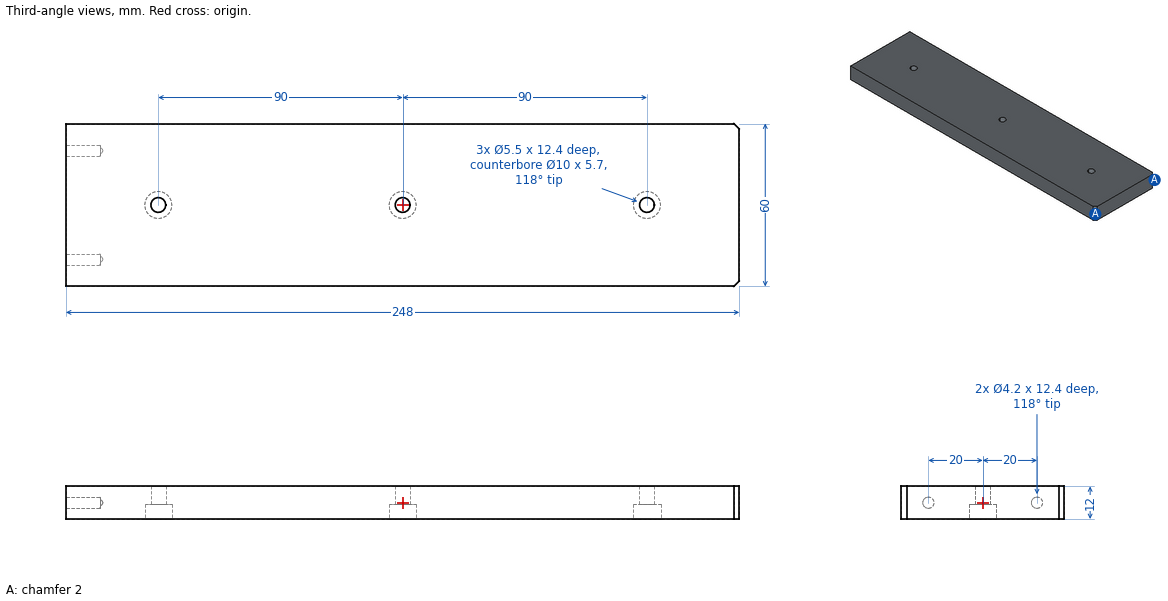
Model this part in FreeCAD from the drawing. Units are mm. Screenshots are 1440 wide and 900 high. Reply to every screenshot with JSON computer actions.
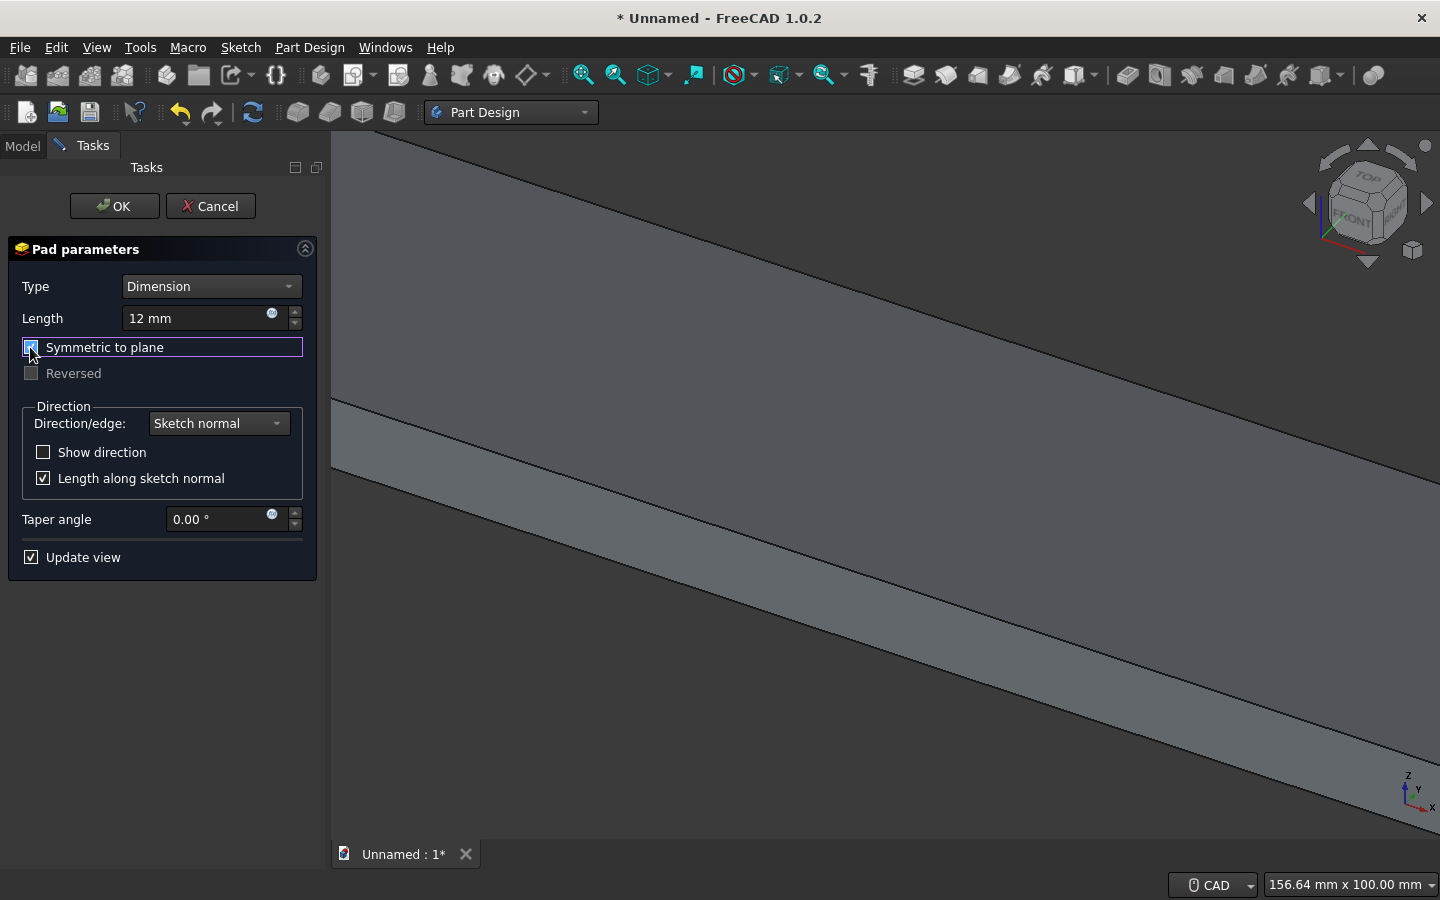
{"action": "left_click", "coordinate": [115, 206]}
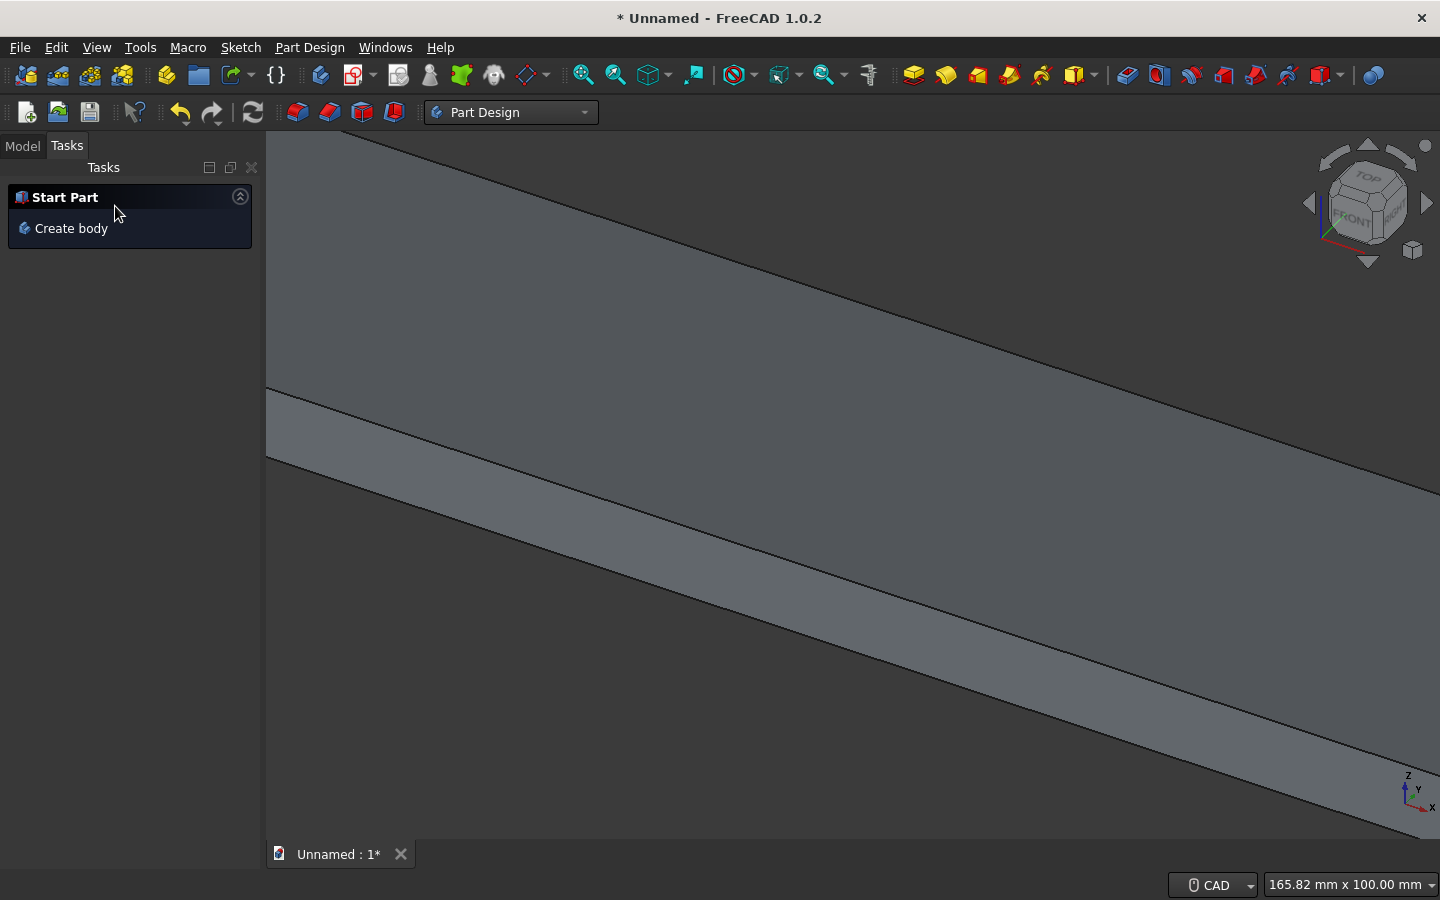
{"action": "left_click", "coordinate": [584, 76]}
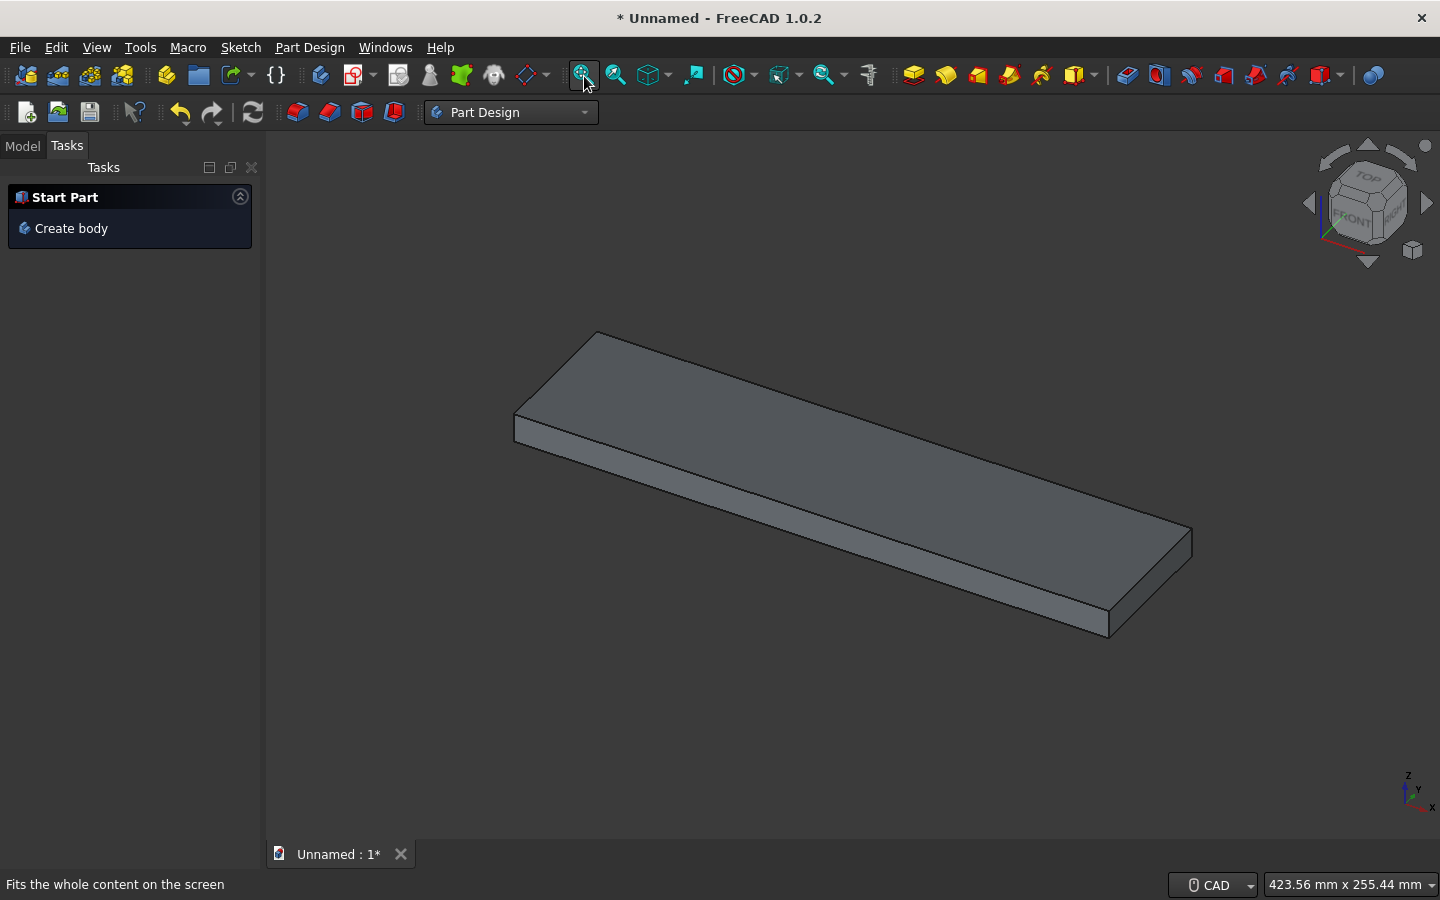
{"action": "key", "text": "6"}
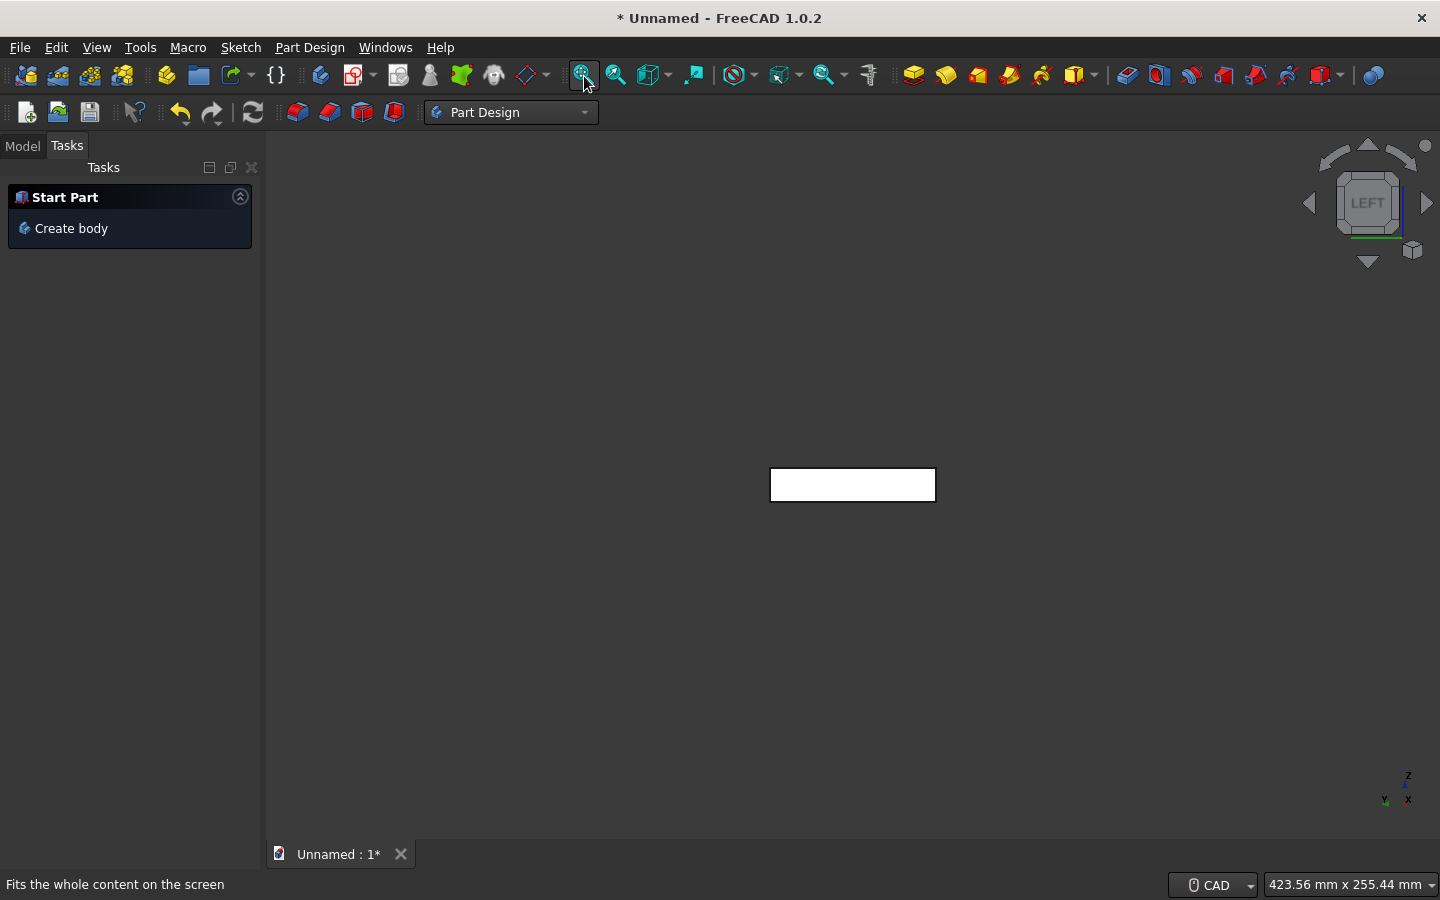
{"action": "left_click", "coordinate": [584, 76]}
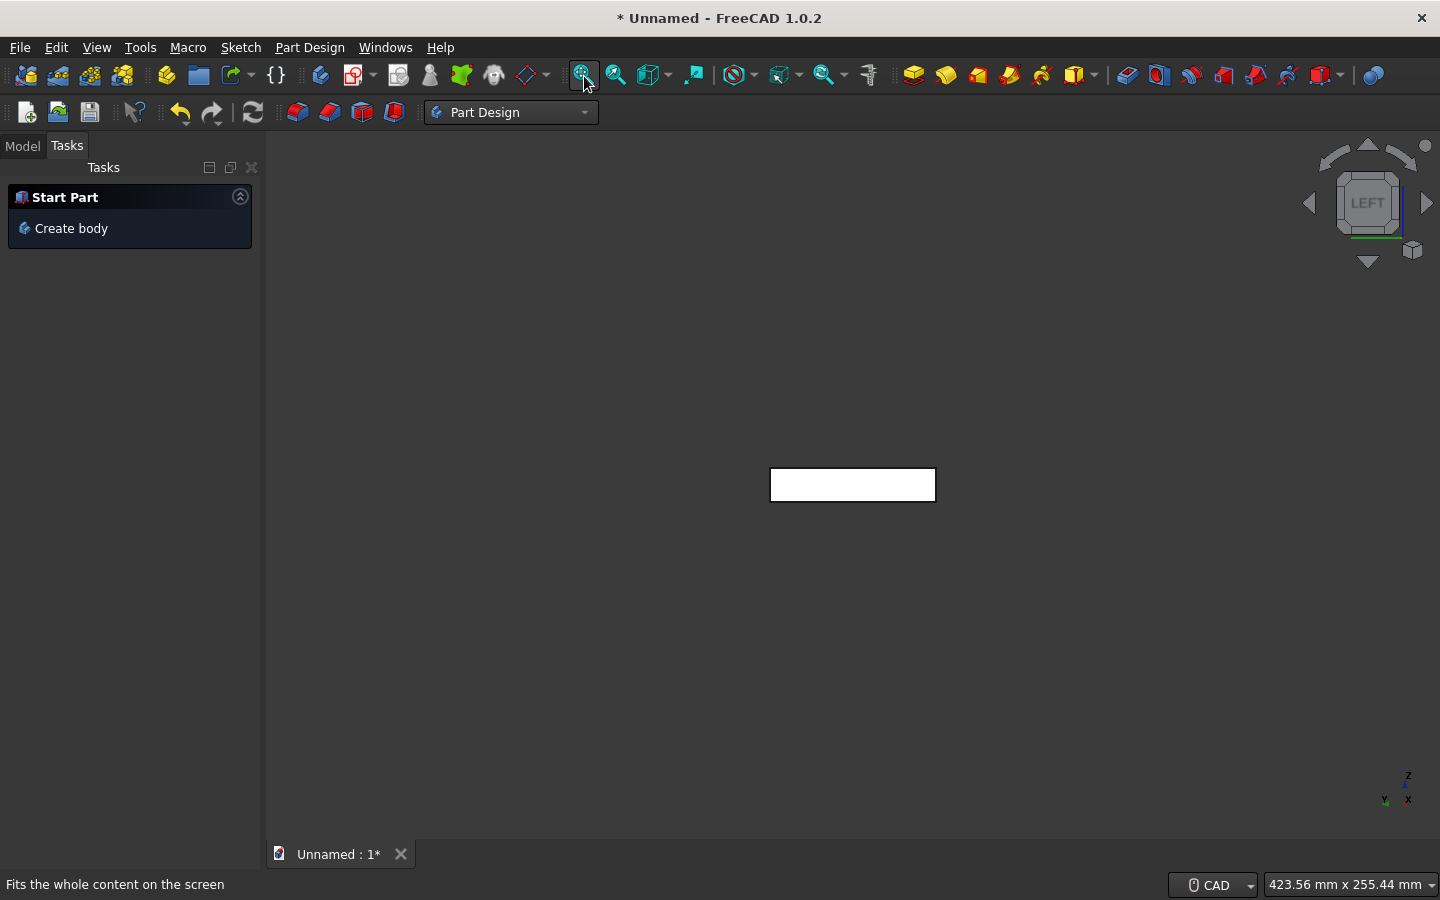
{"action": "left_click", "coordinate": [805, 484]}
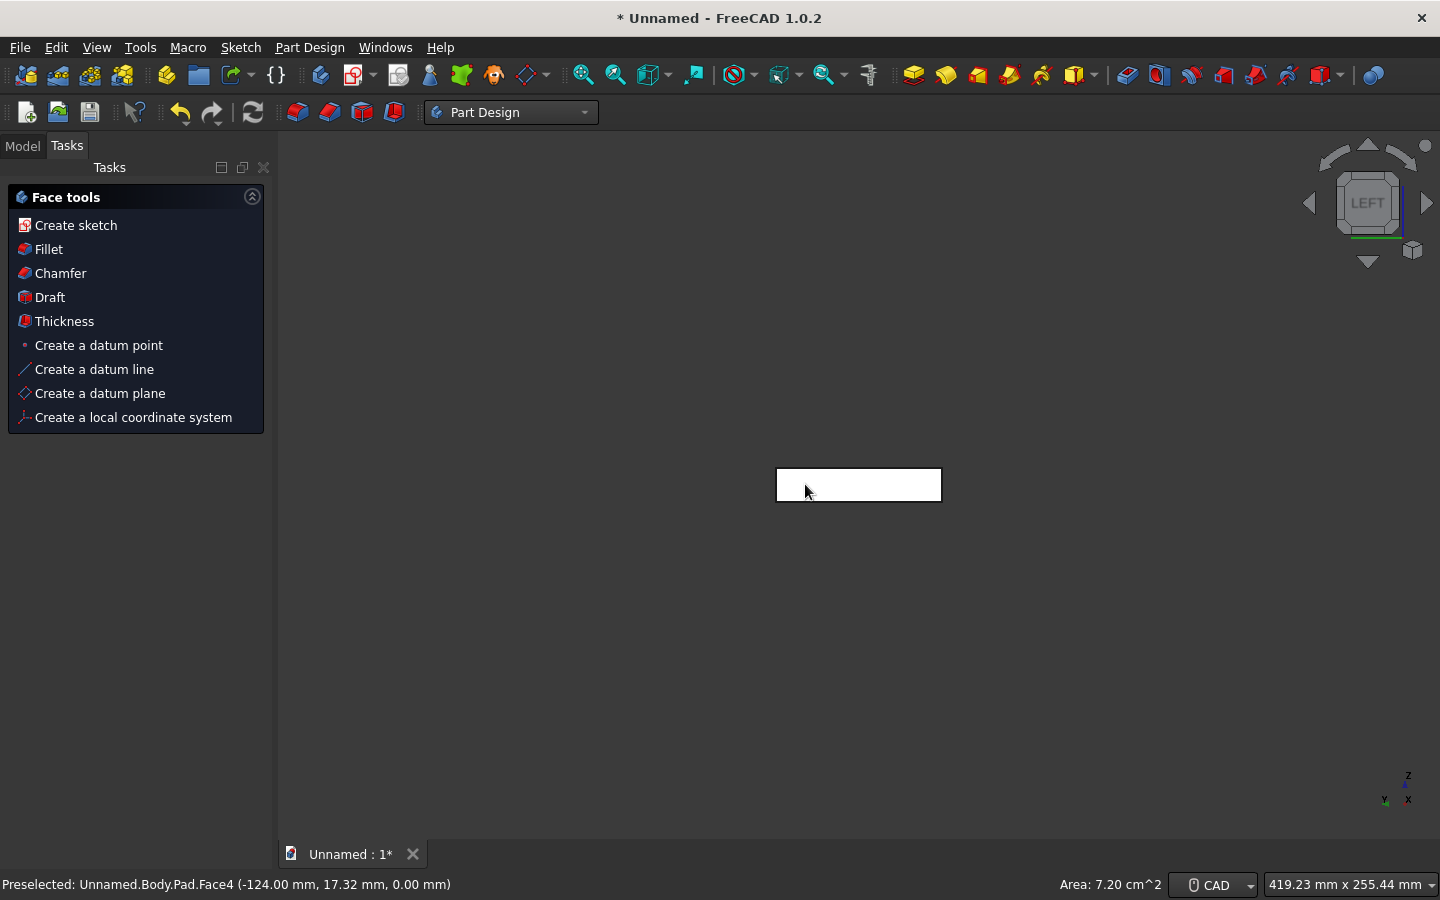
{"action": "left_click", "coordinate": [354, 76]}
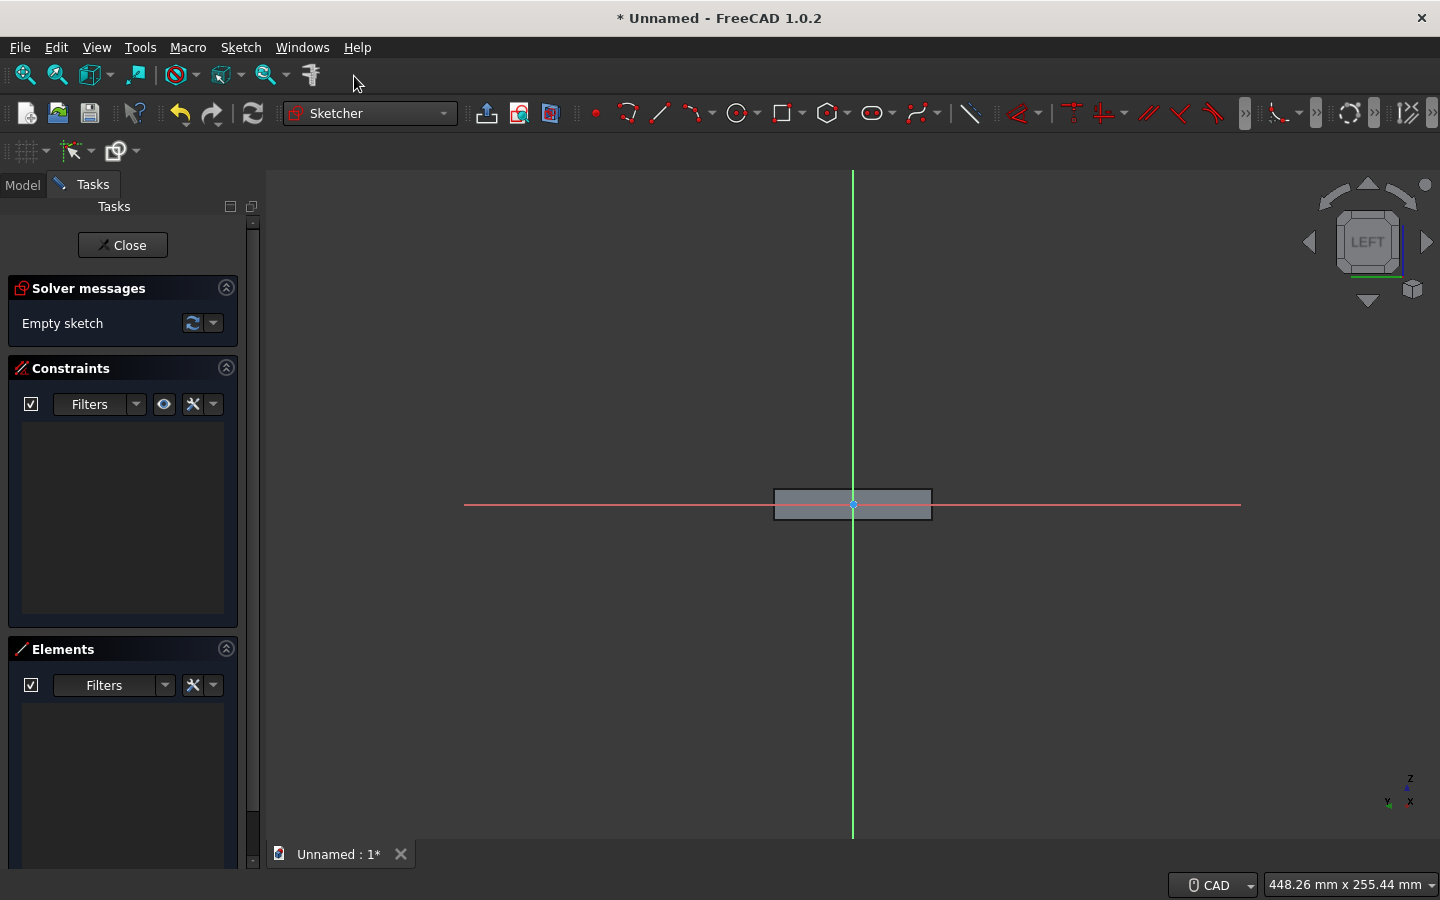
{"action": "scroll", "coordinate": [867, 505], "scroll_direction": "up", "scroll_amount": 9}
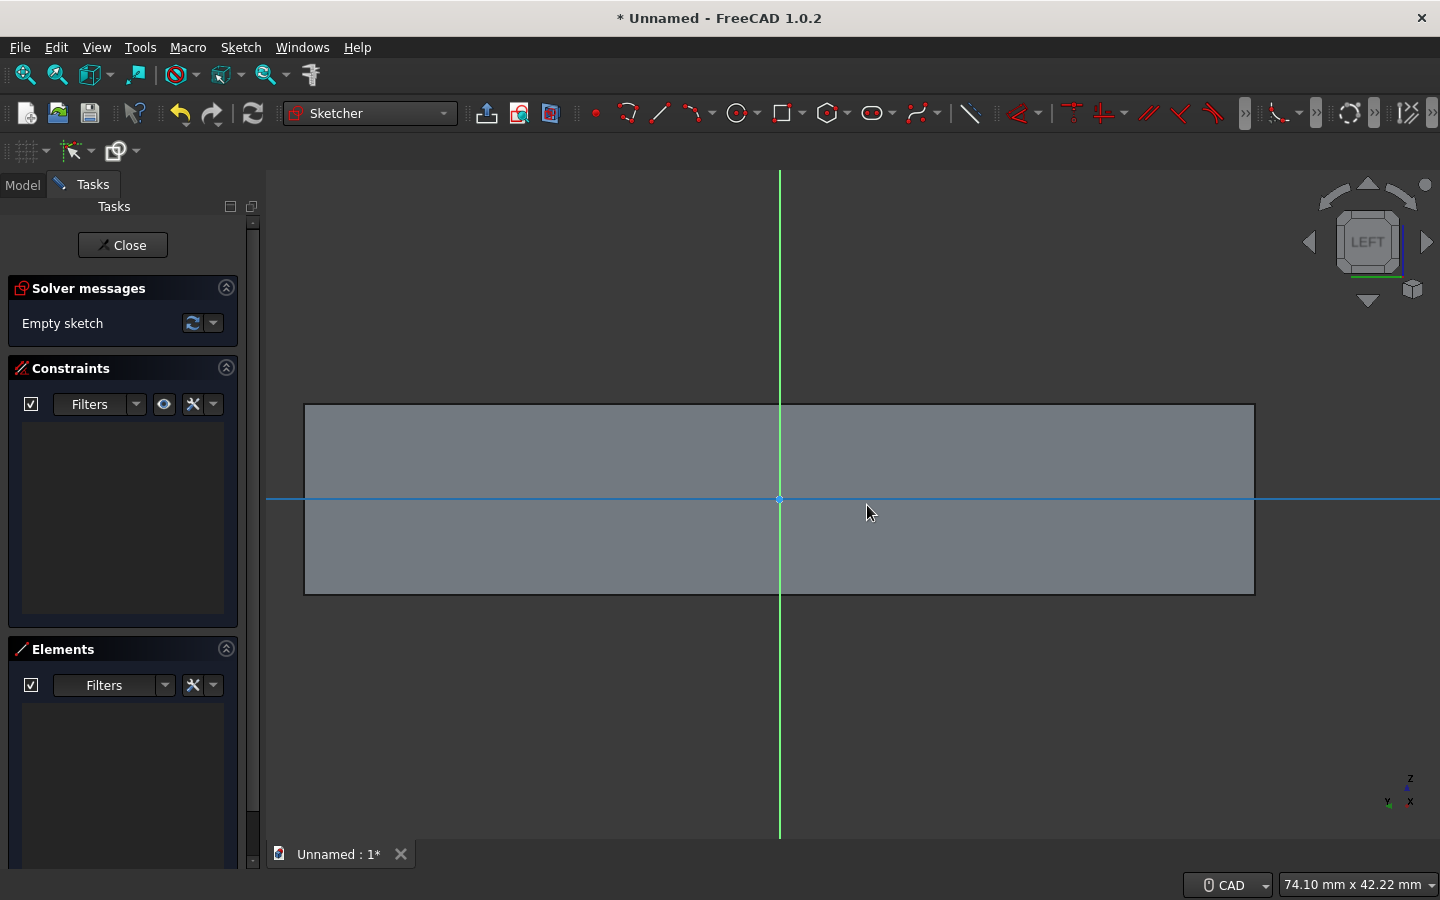
{"action": "left_click", "coordinate": [738, 114]}